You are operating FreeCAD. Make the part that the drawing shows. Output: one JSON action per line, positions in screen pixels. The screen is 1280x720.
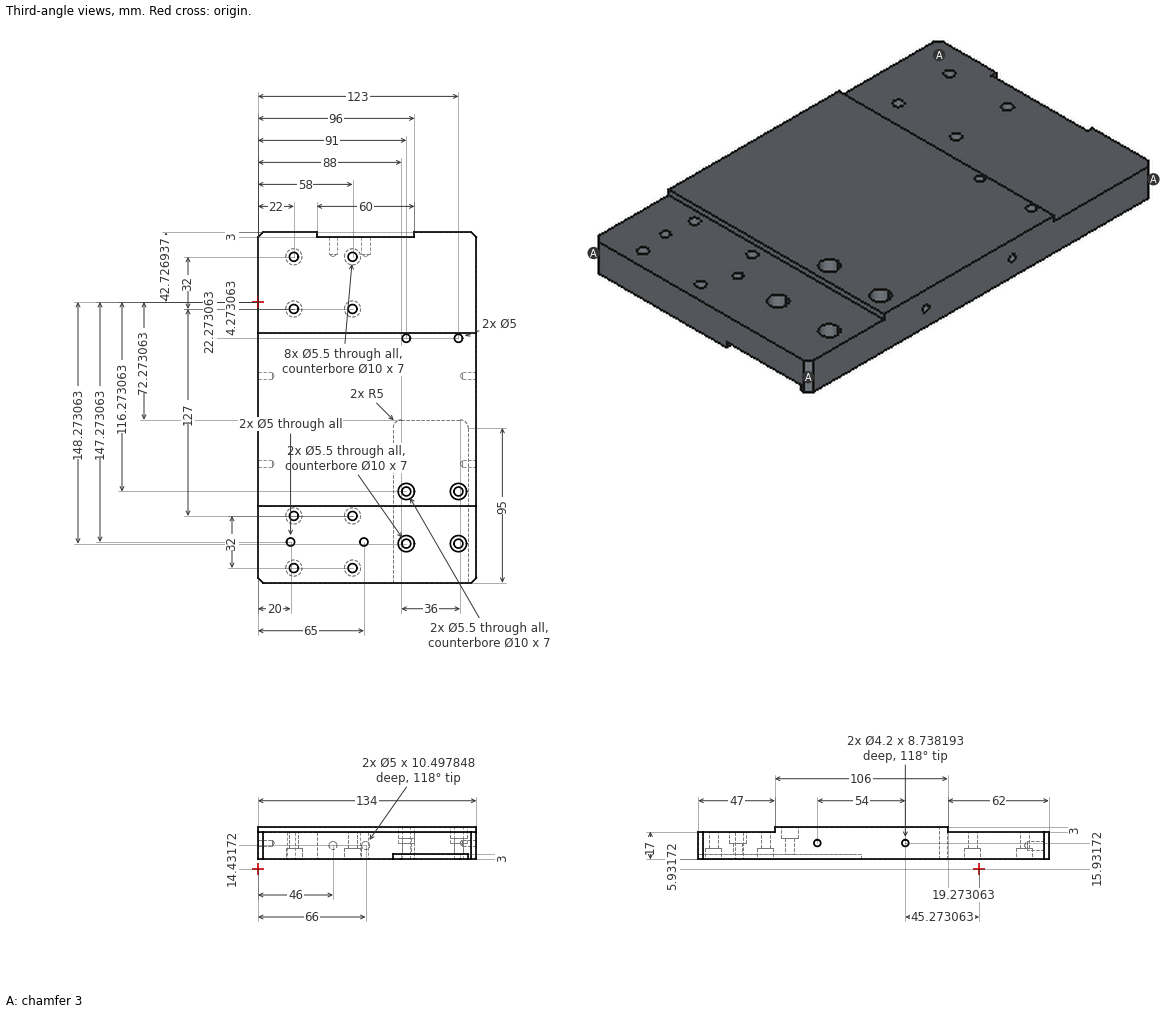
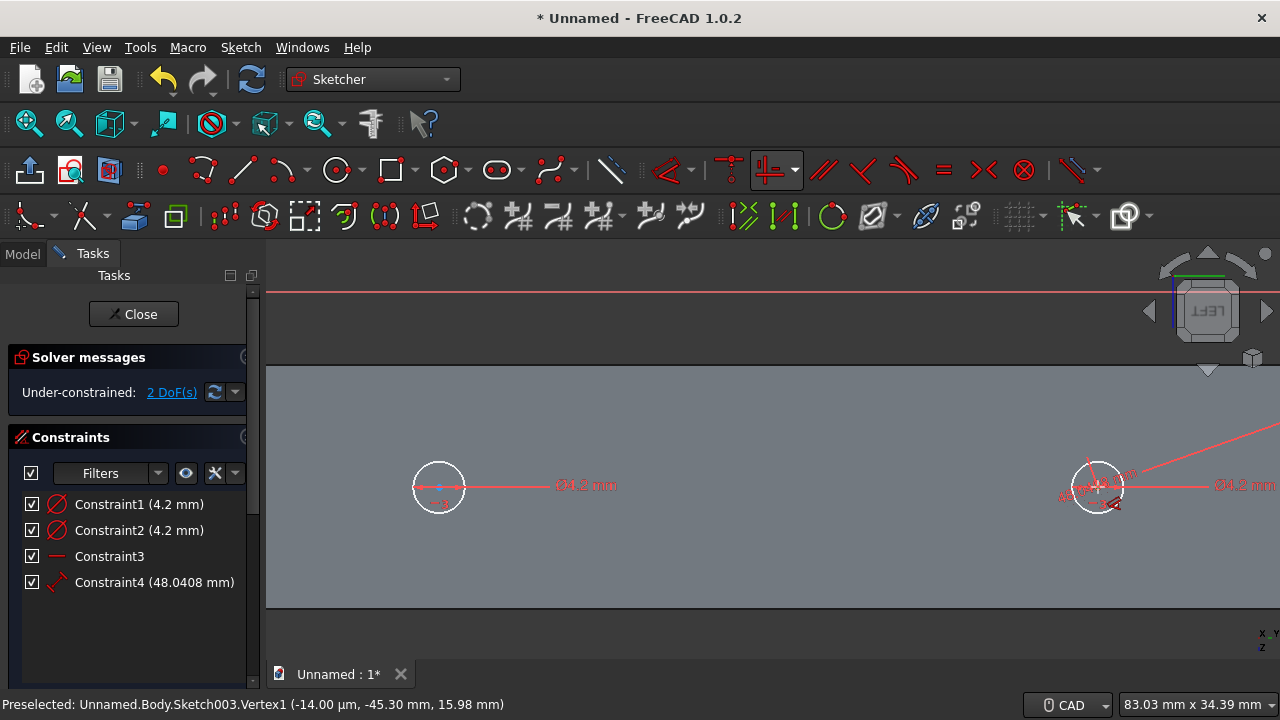
{"action": "left_click", "coordinate": [439, 487]}
{"action": "left_click", "coordinate": [768, 521]}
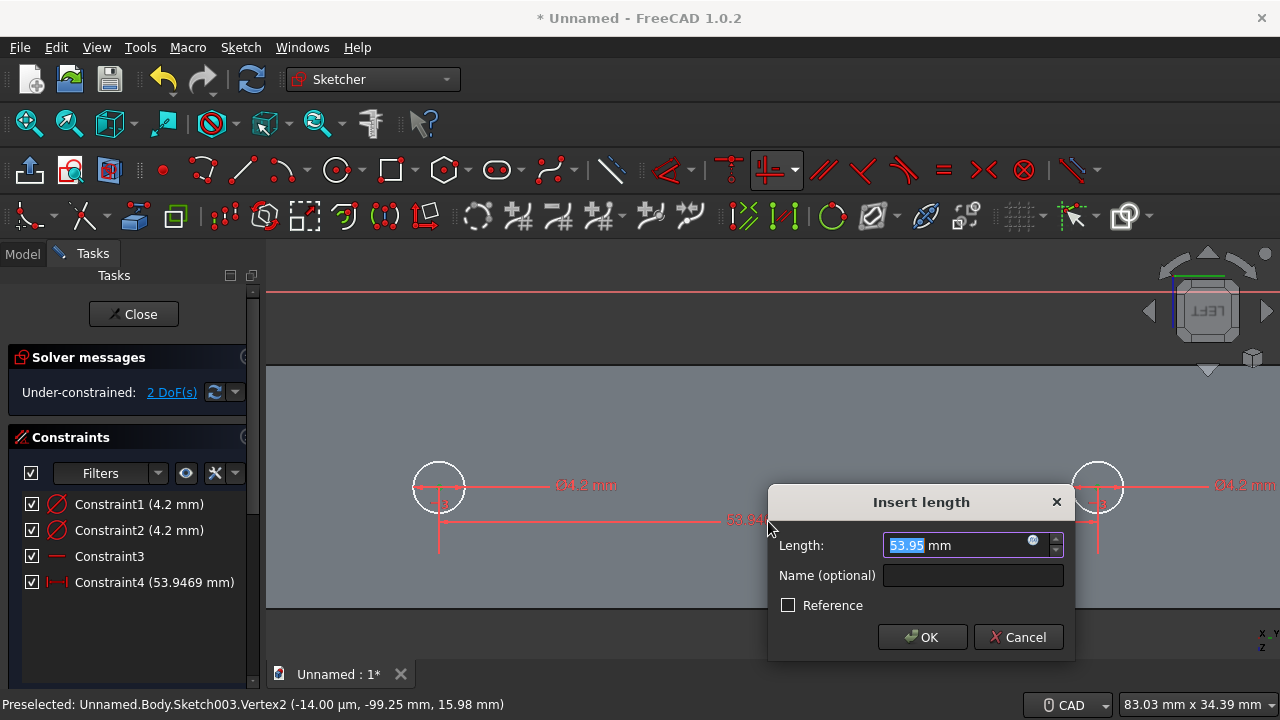
{"action": "type", "text": "54"}
{"action": "key", "text": "Return"}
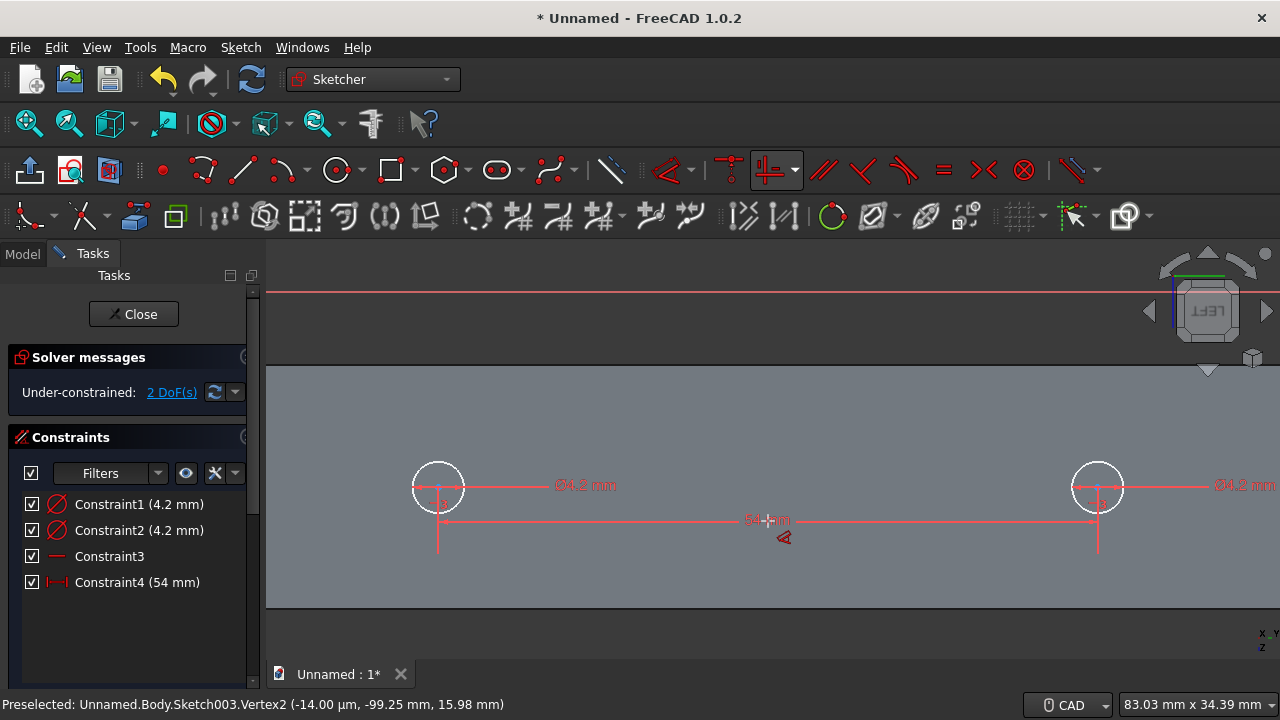
{"action": "left_click", "coordinate": [1098, 487]}
{"action": "left_click", "coordinate": [1064, 390]}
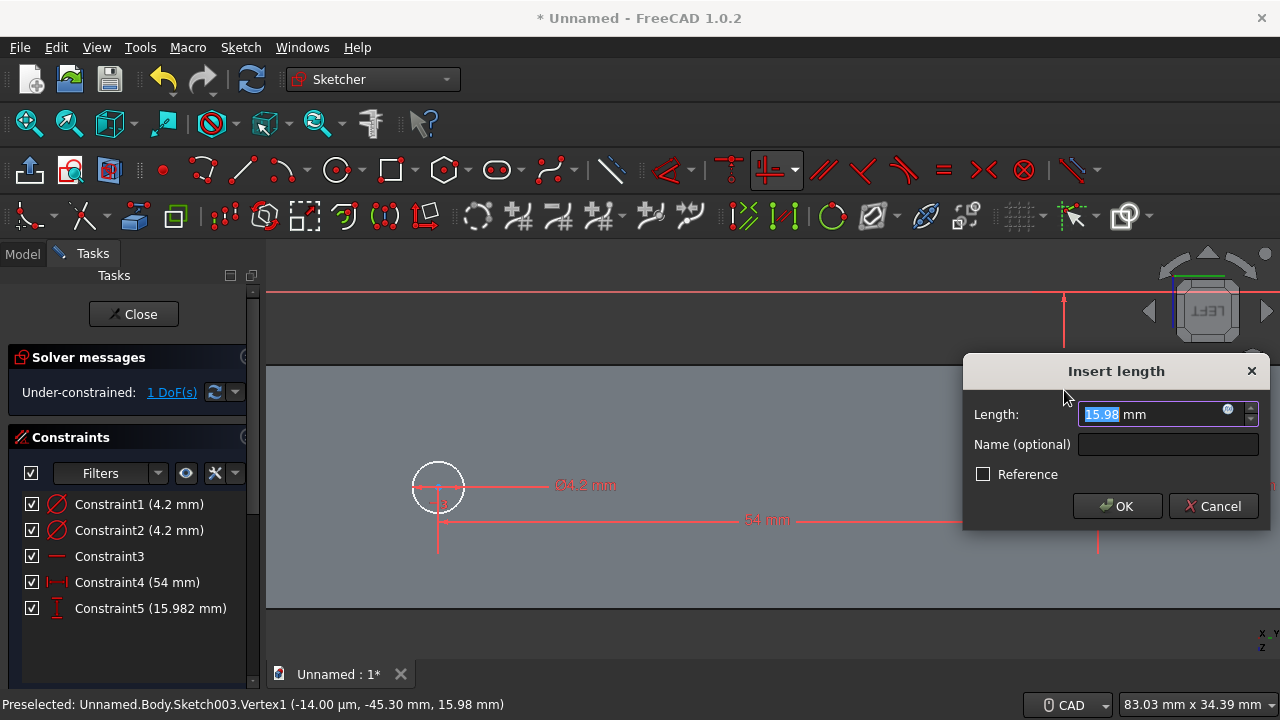
{"action": "type", "text": "15.93172"}
{"action": "key", "text": "Return"}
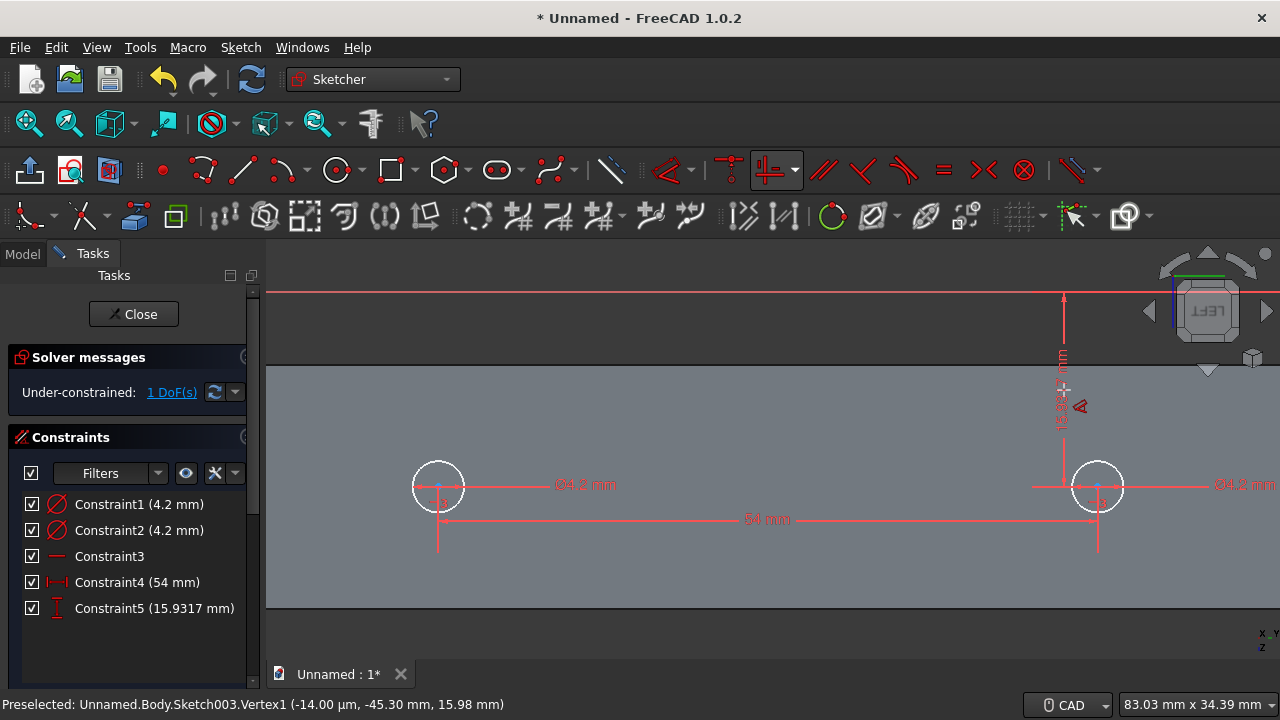
{"action": "left_click", "coordinate": [1098, 487]}
{"action": "left_click", "coordinate": [1106, 545]}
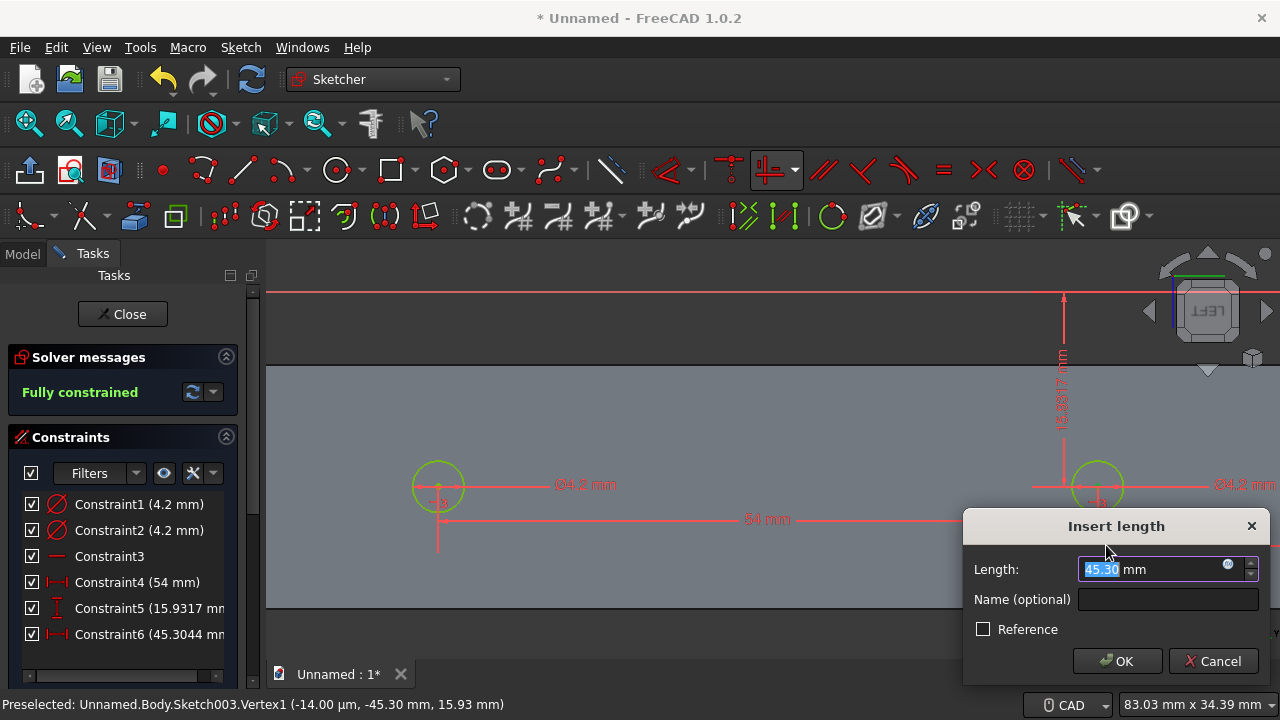
{"action": "type", "text": "45.273063"}
{"action": "key", "text": "Return"}
{"action": "key", "text": "Escape"}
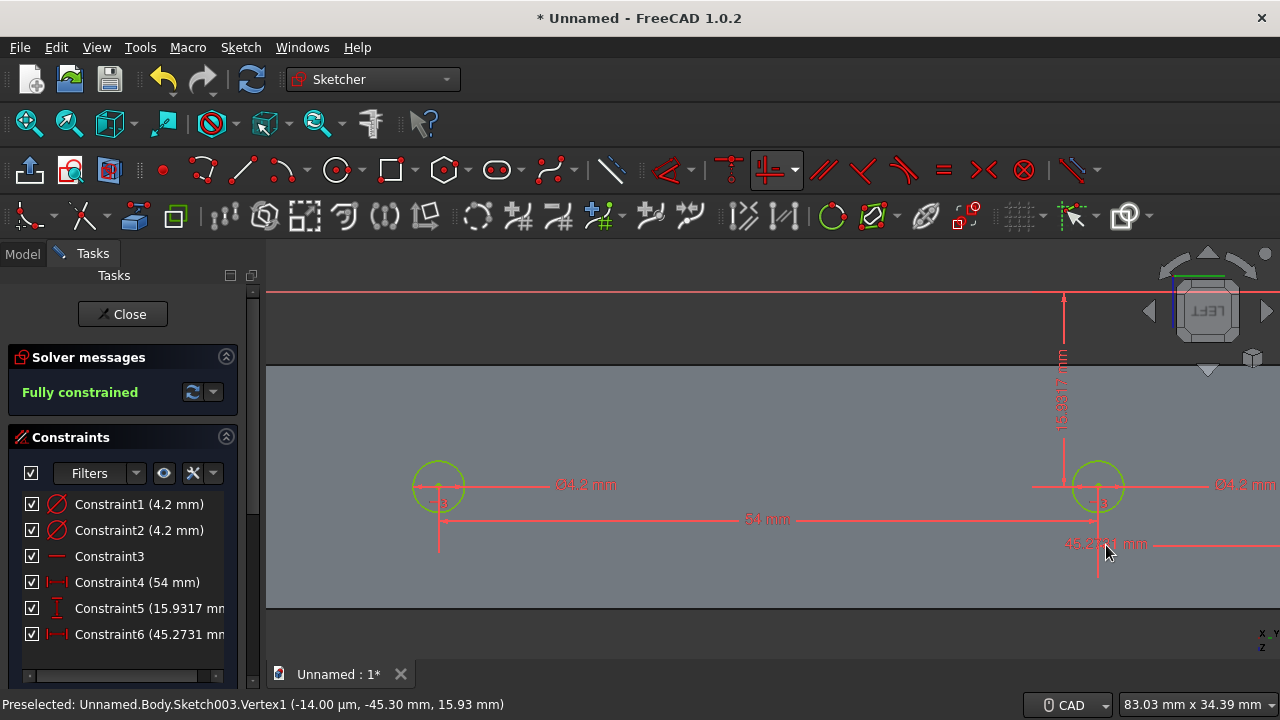
{"action": "left_click", "coordinate": [123, 314]}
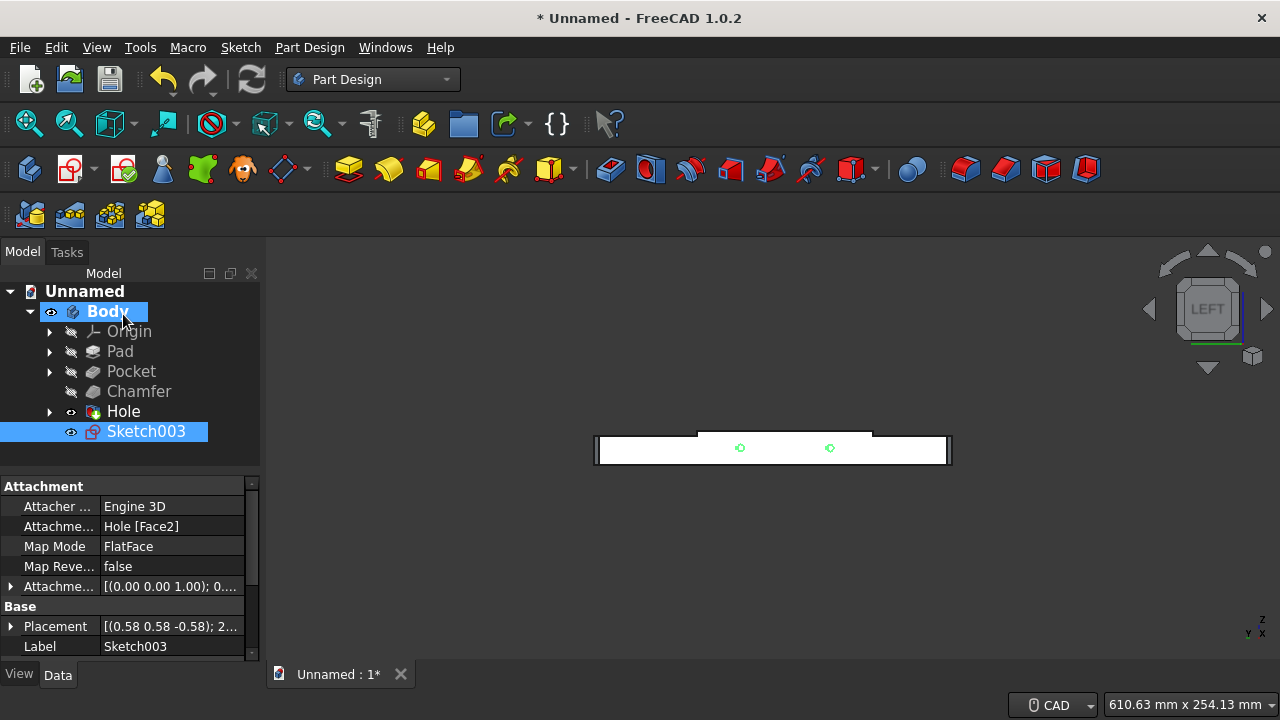
{"action": "left_click", "coordinate": [652, 170]}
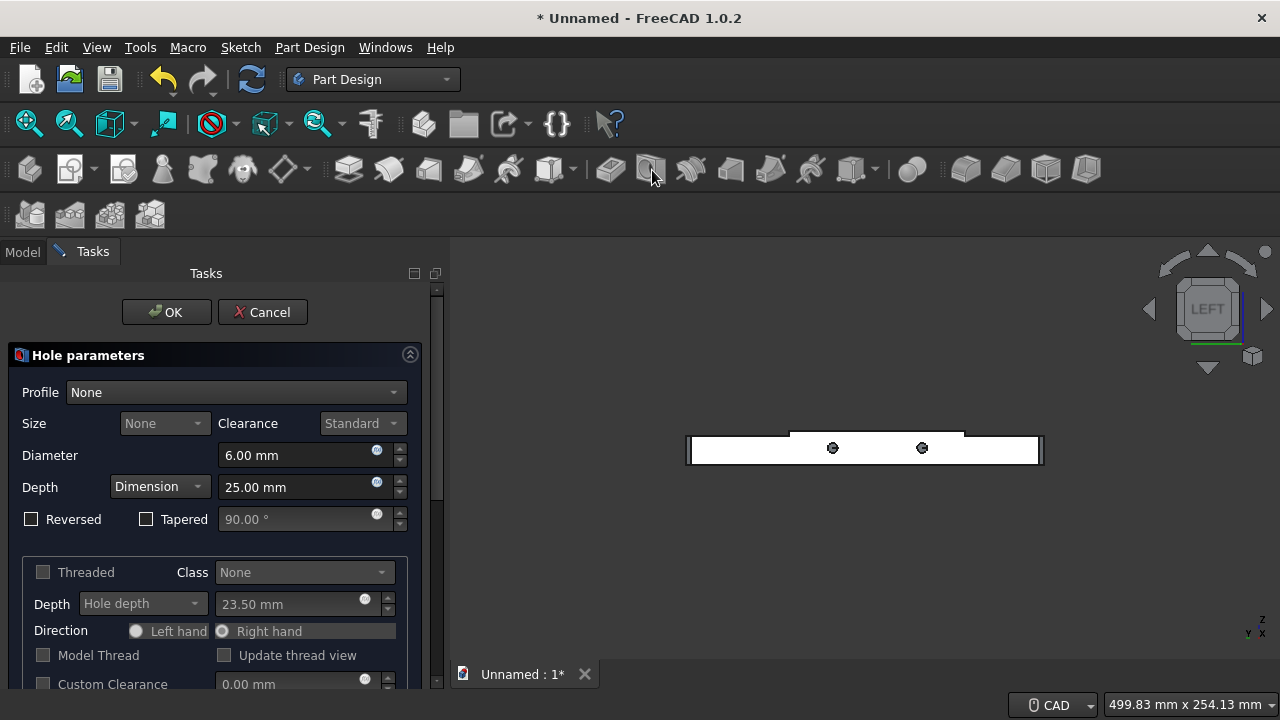
{"action": "triple_click", "coordinate": [305, 455]}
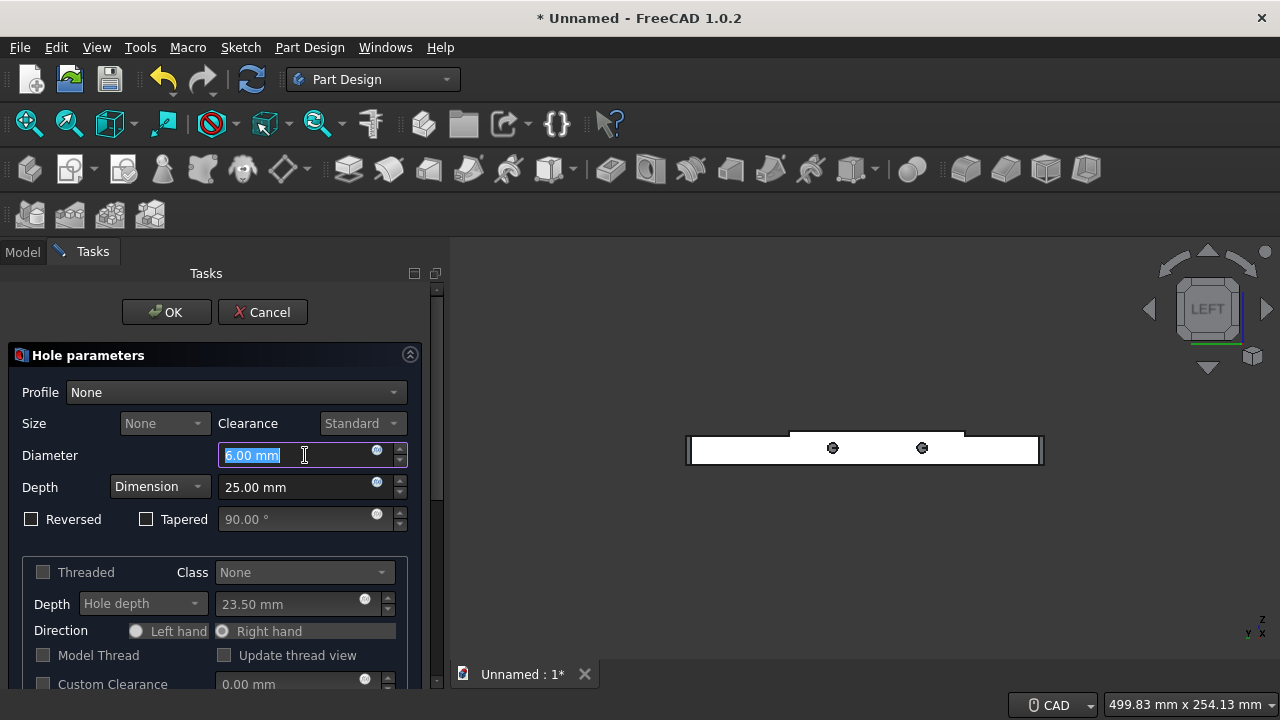
{"action": "type", "text": "4.2"}
{"action": "key", "text": "Tab"}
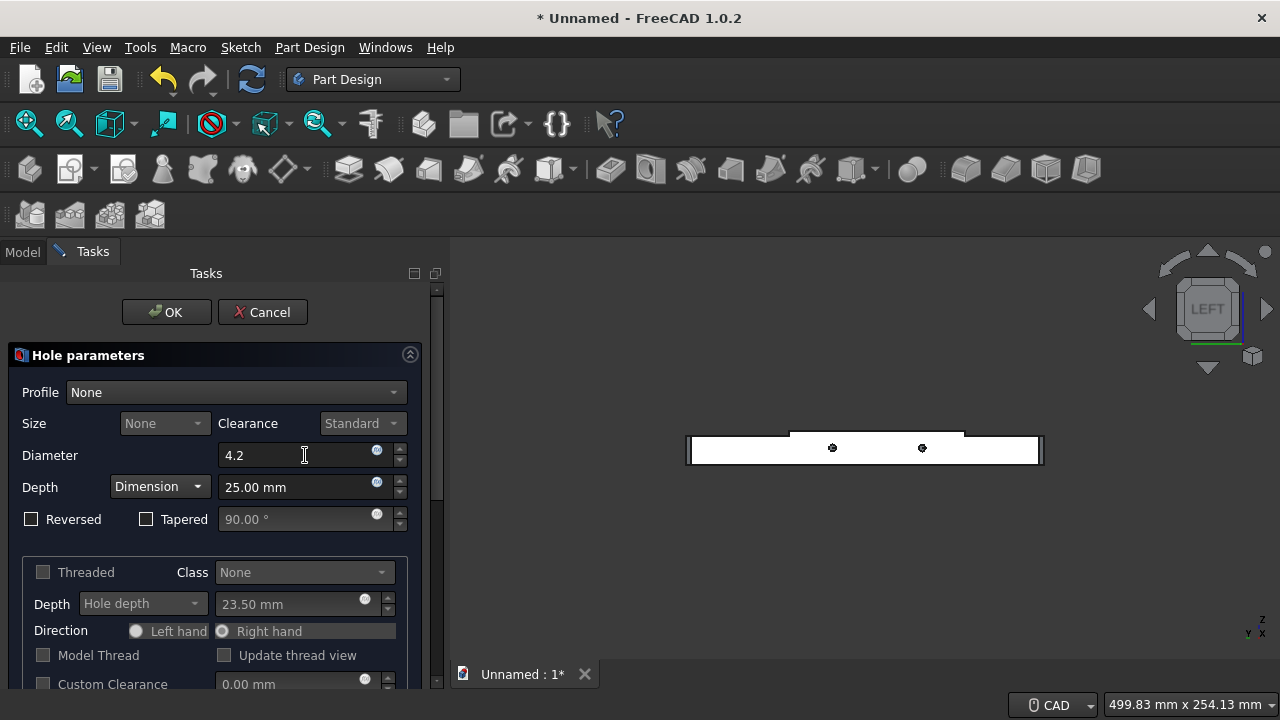
{"action": "triple_click", "coordinate": [305, 487]}